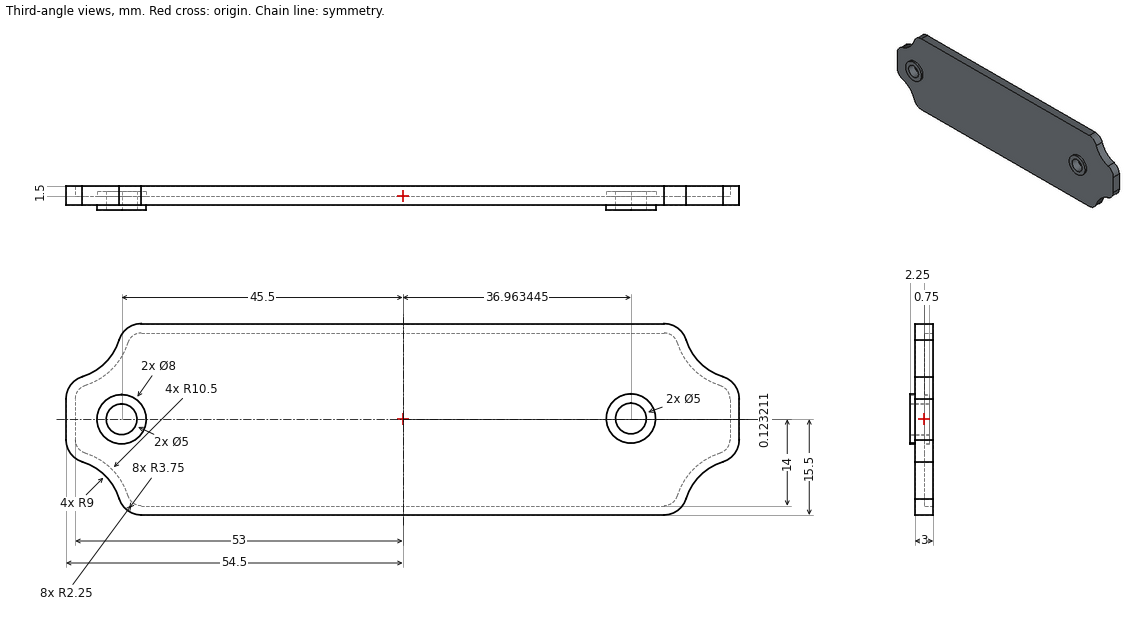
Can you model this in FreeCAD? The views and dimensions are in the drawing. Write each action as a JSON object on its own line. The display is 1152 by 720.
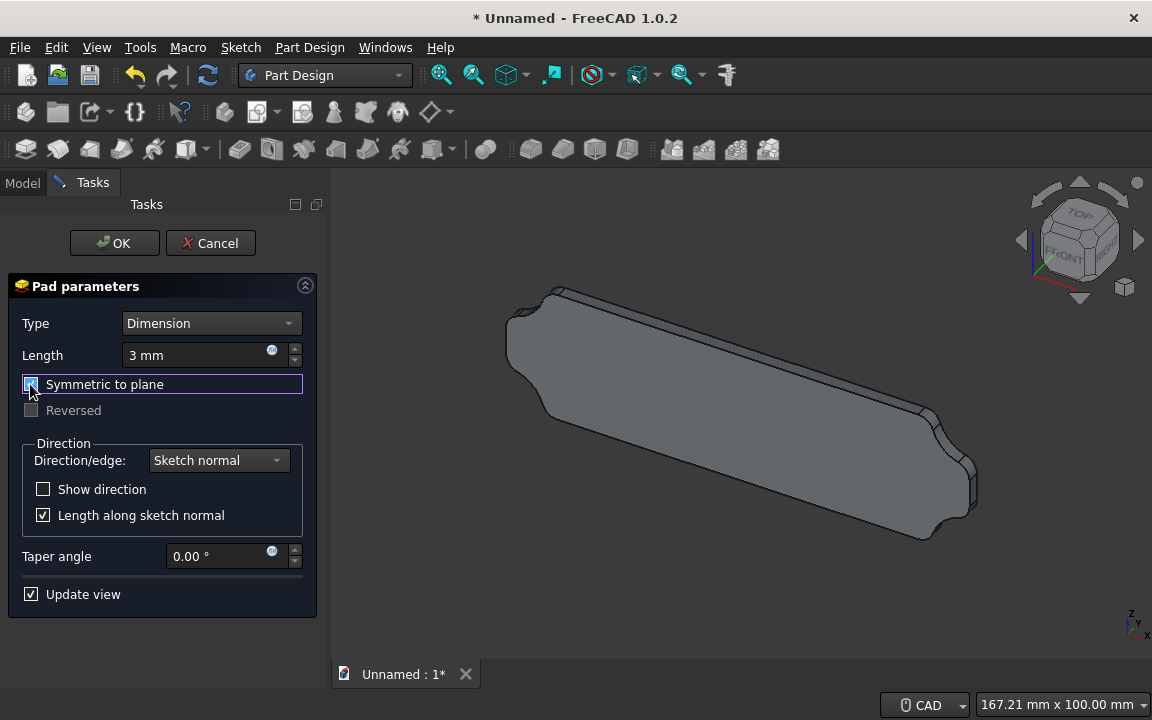
{"action": "left_click", "coordinate": [115, 243]}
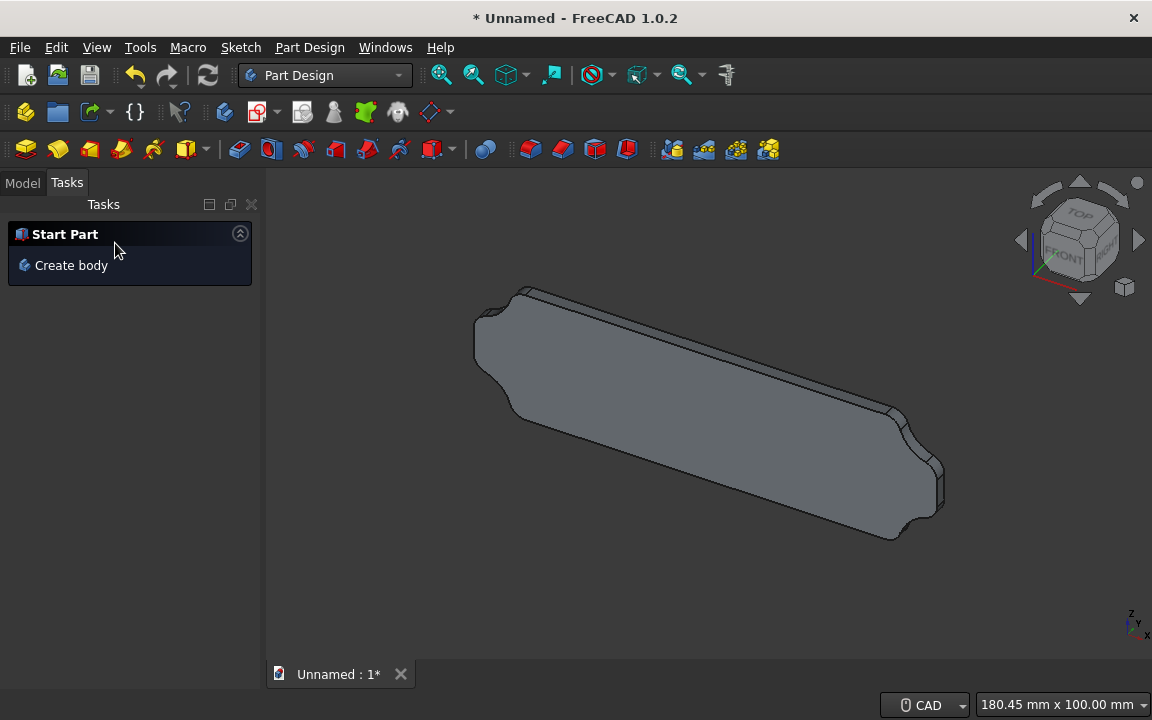
{"action": "key", "text": "4"}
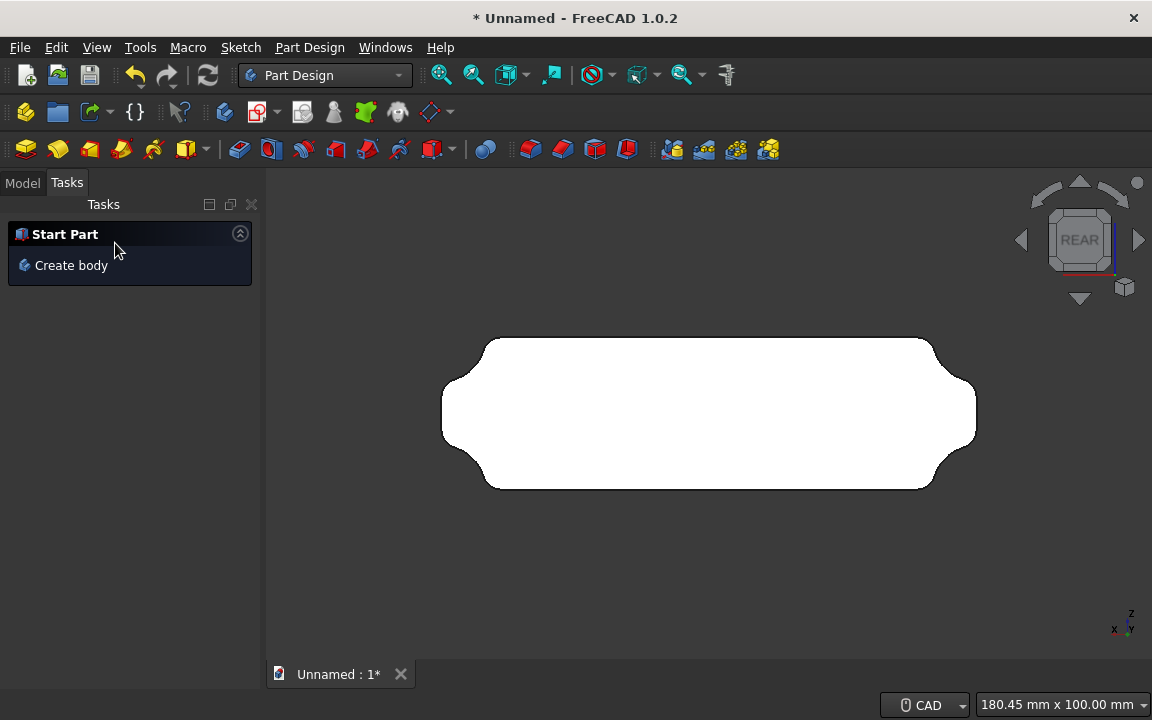
{"action": "left_click", "coordinate": [556, 412]}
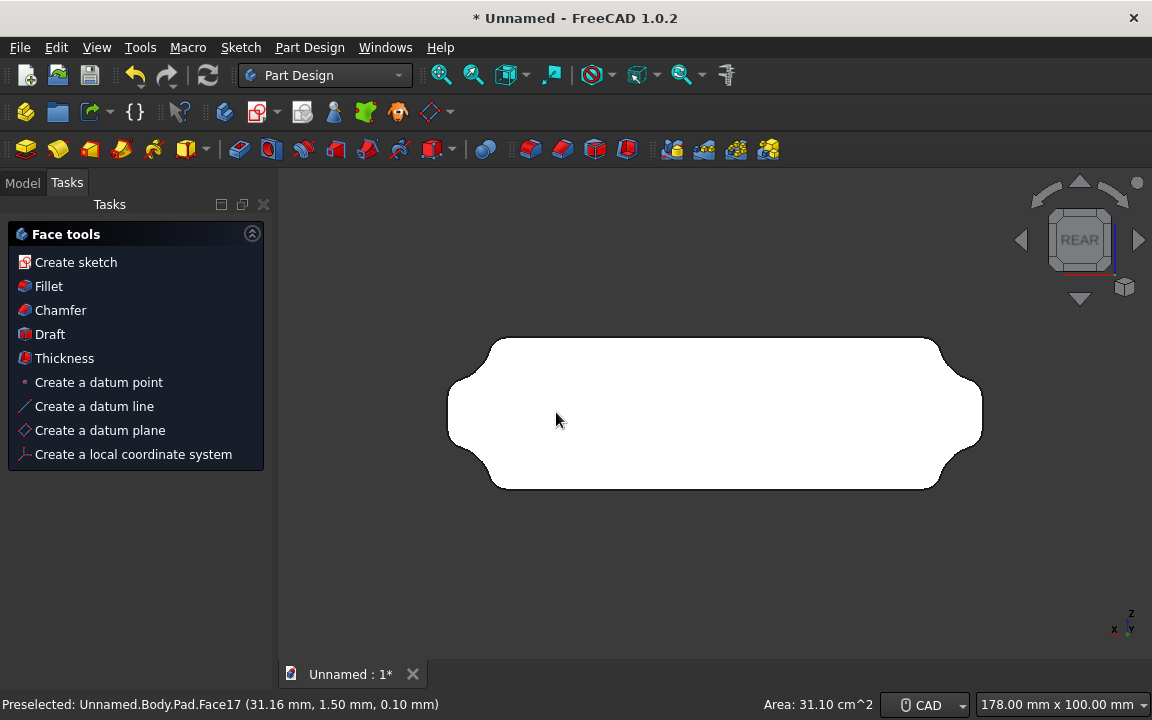
{"action": "left_click", "coordinate": [258, 112]}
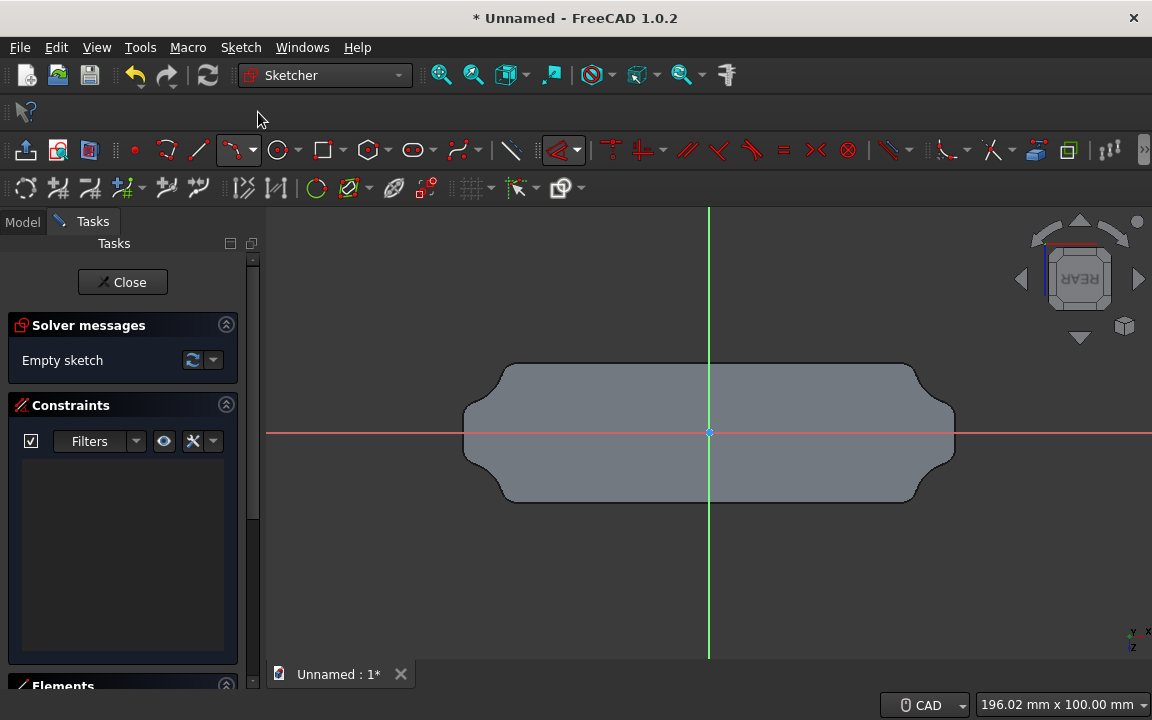
{"action": "left_click", "coordinate": [200, 150]}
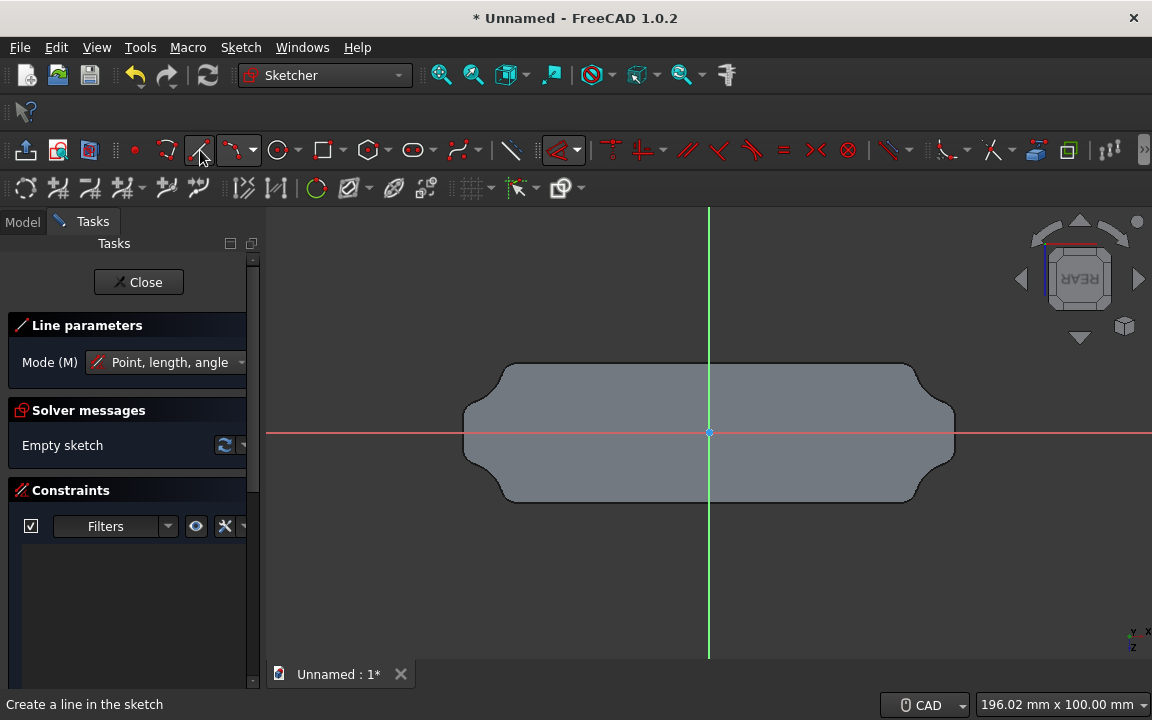
{"action": "left_click", "coordinate": [900, 370]}
{"action": "left_click", "coordinate": [518, 370]}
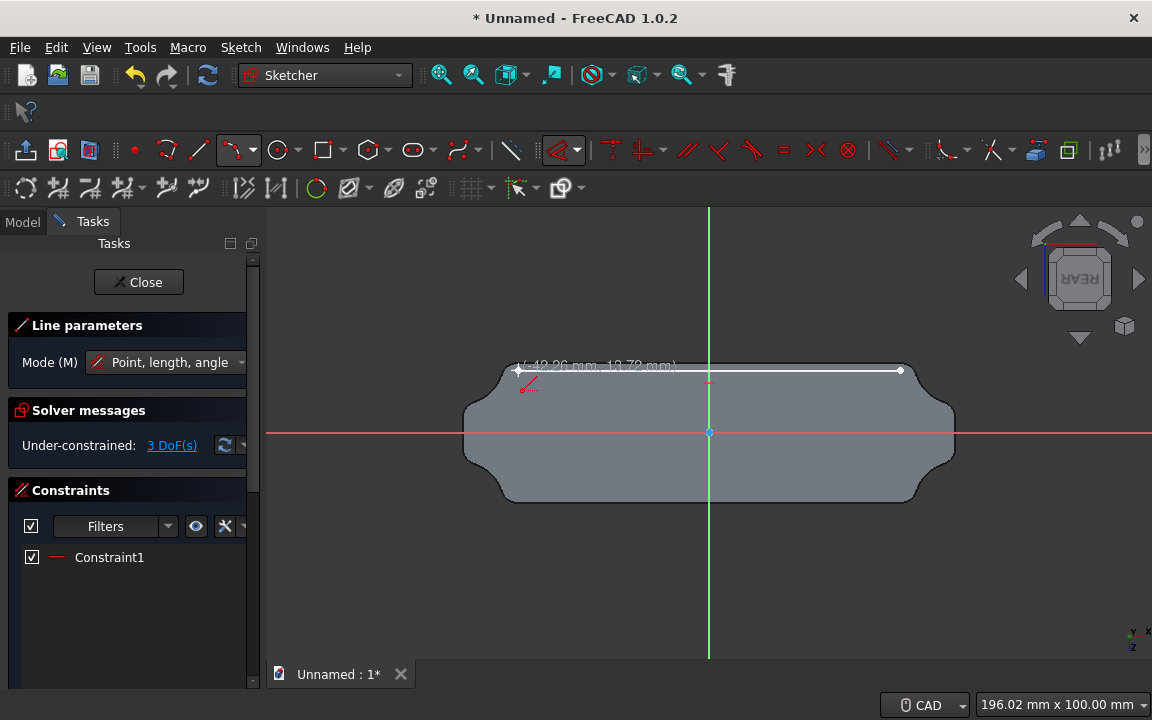
{"action": "left_click", "coordinate": [469, 418]}
{"action": "left_click", "coordinate": [469, 448]}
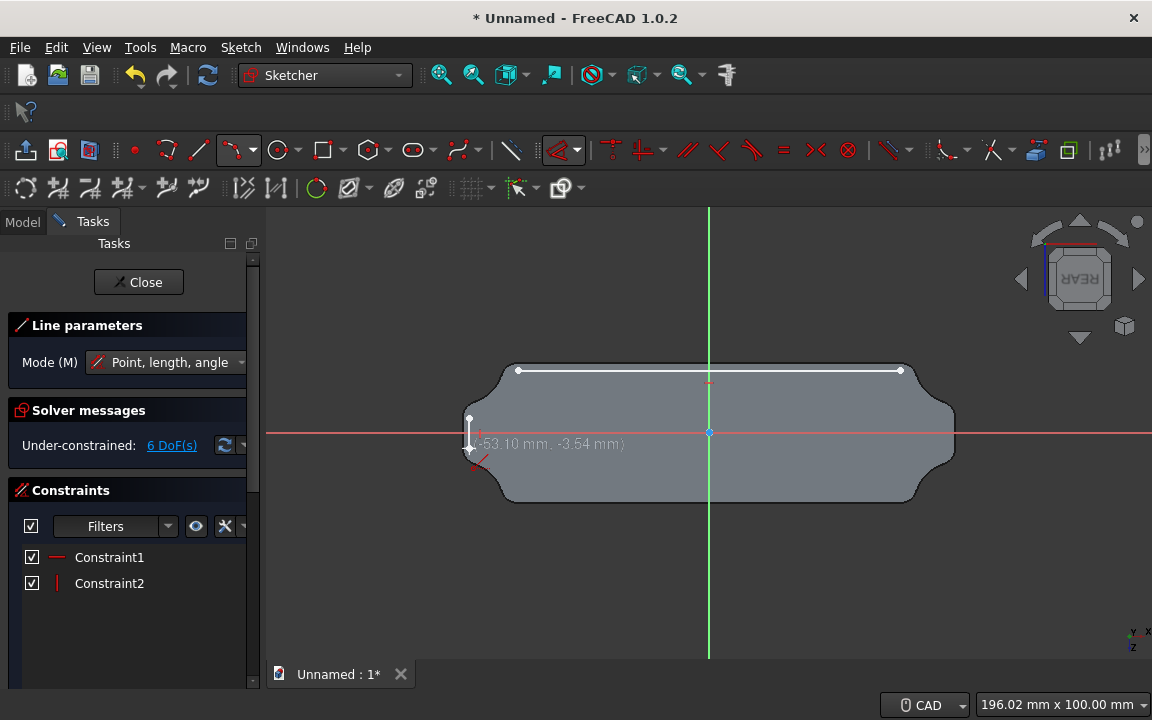
{"action": "left_click", "coordinate": [518, 496]}
{"action": "left_click", "coordinate": [900, 496]}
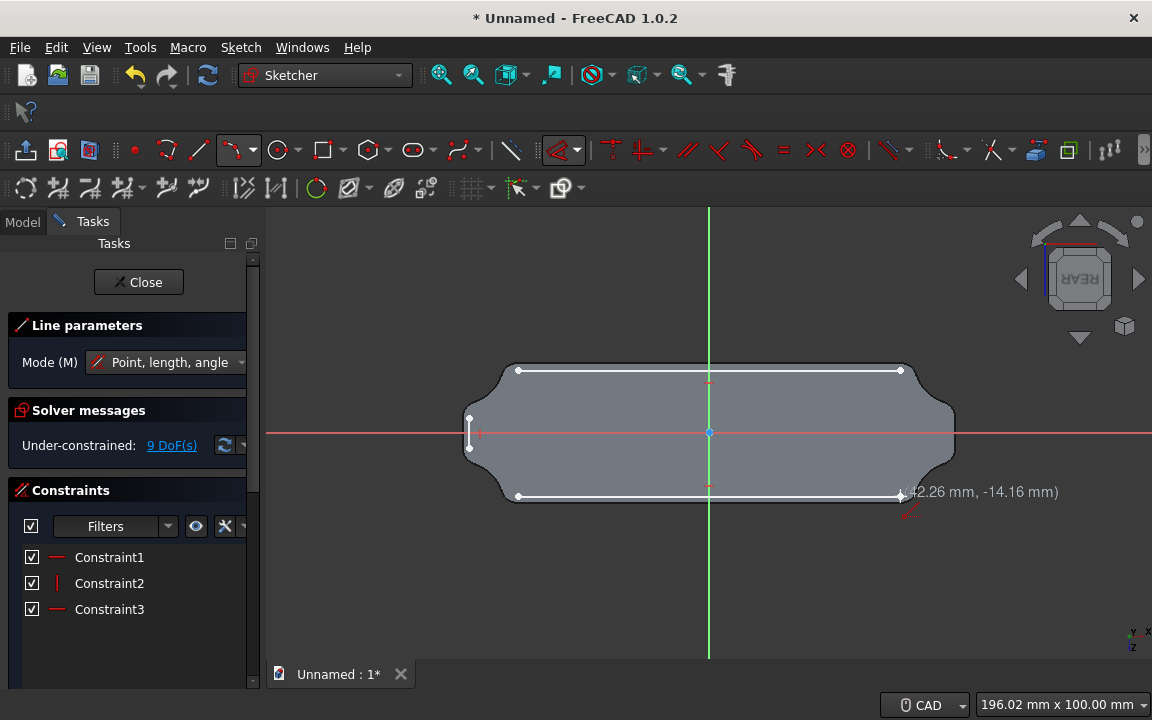
{"action": "left_click", "coordinate": [949, 448]}
{"action": "left_click", "coordinate": [949, 418]}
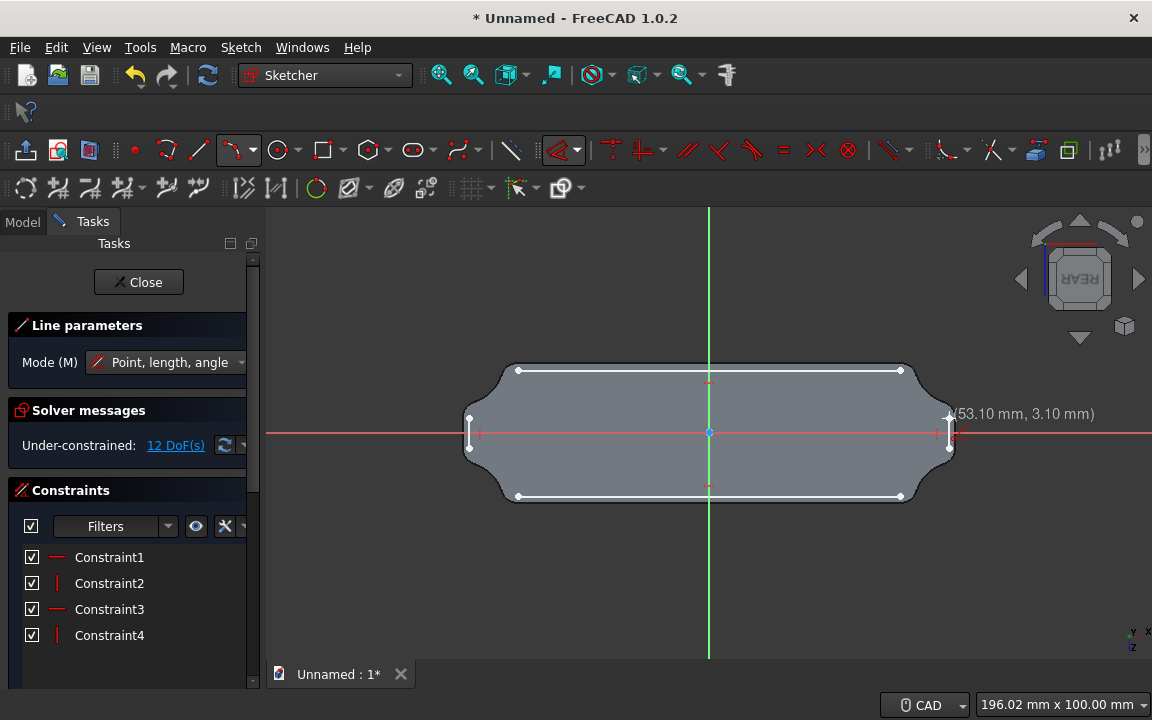
{"action": "left_click", "coordinate": [232, 150]}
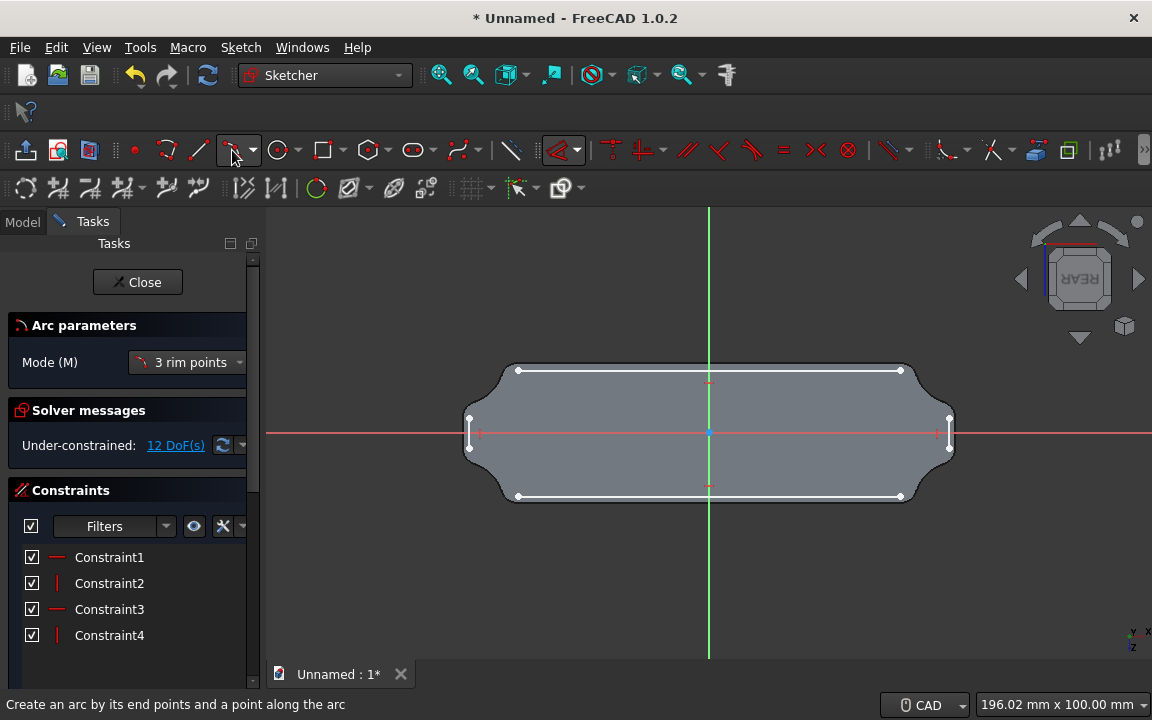
{"action": "left_click", "coordinate": [518, 371]}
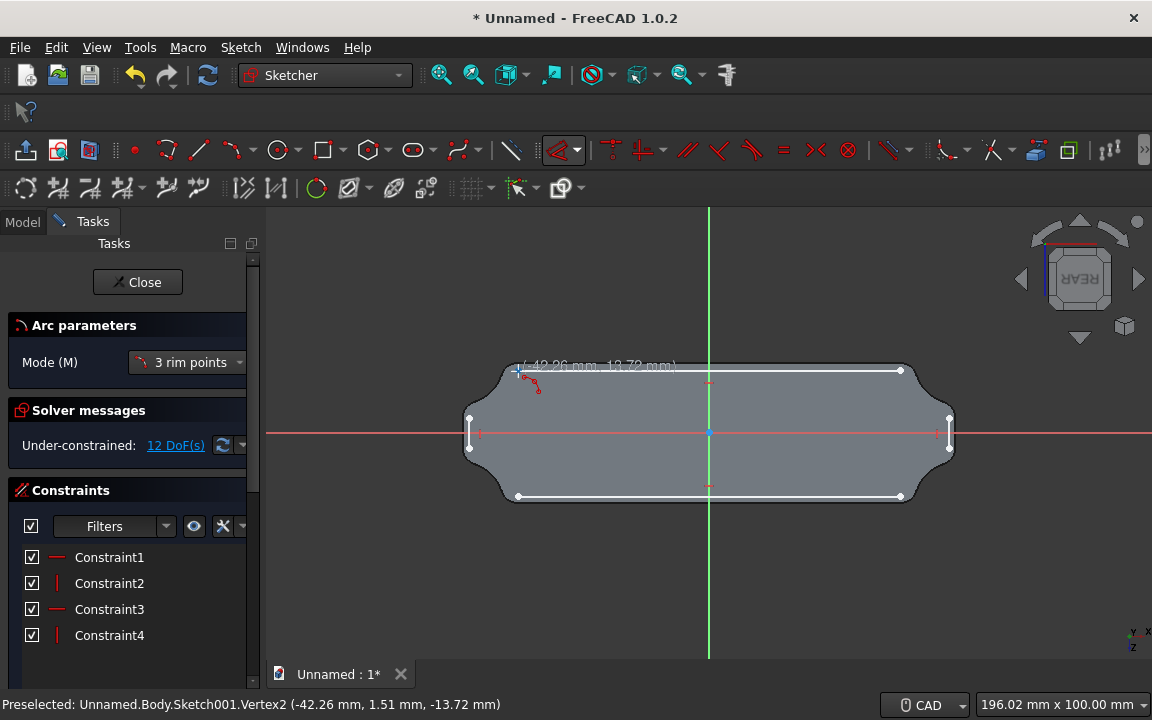
{"action": "scroll", "coordinate": [508, 377], "scroll_direction": "up", "scroll_amount": 2}